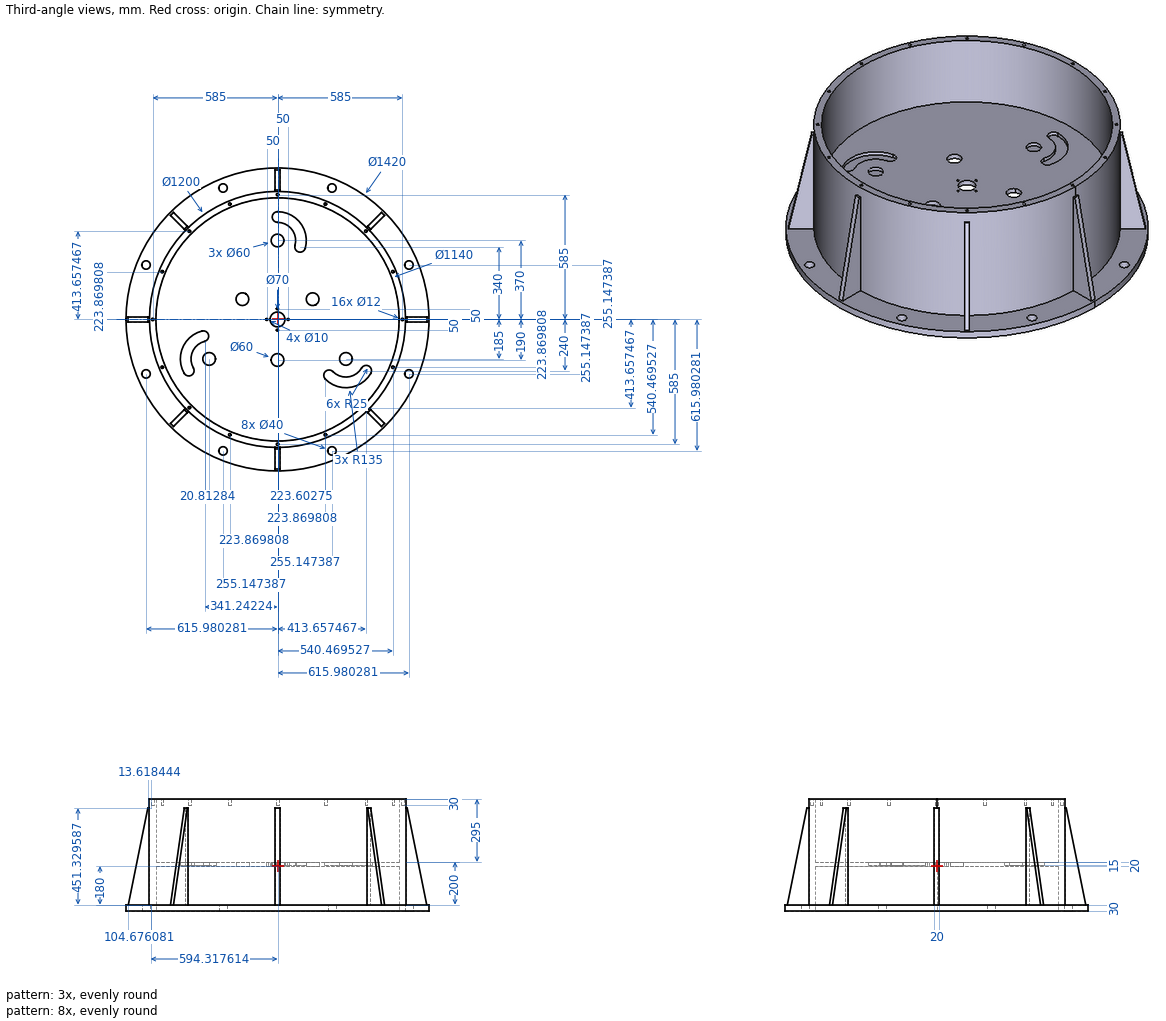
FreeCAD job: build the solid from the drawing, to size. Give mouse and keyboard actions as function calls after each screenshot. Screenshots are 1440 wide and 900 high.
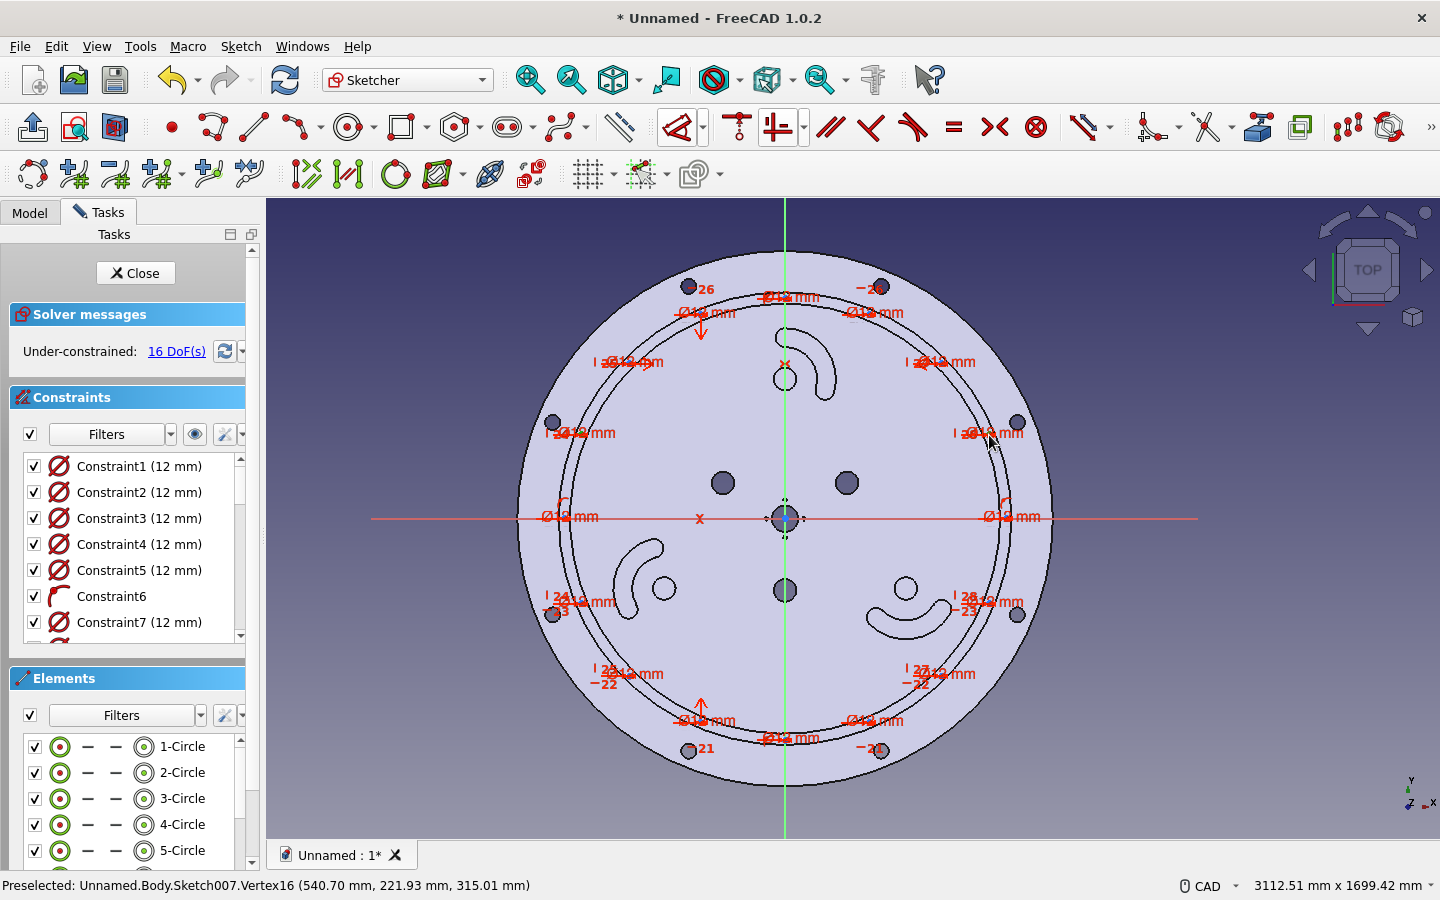
click(785, 686)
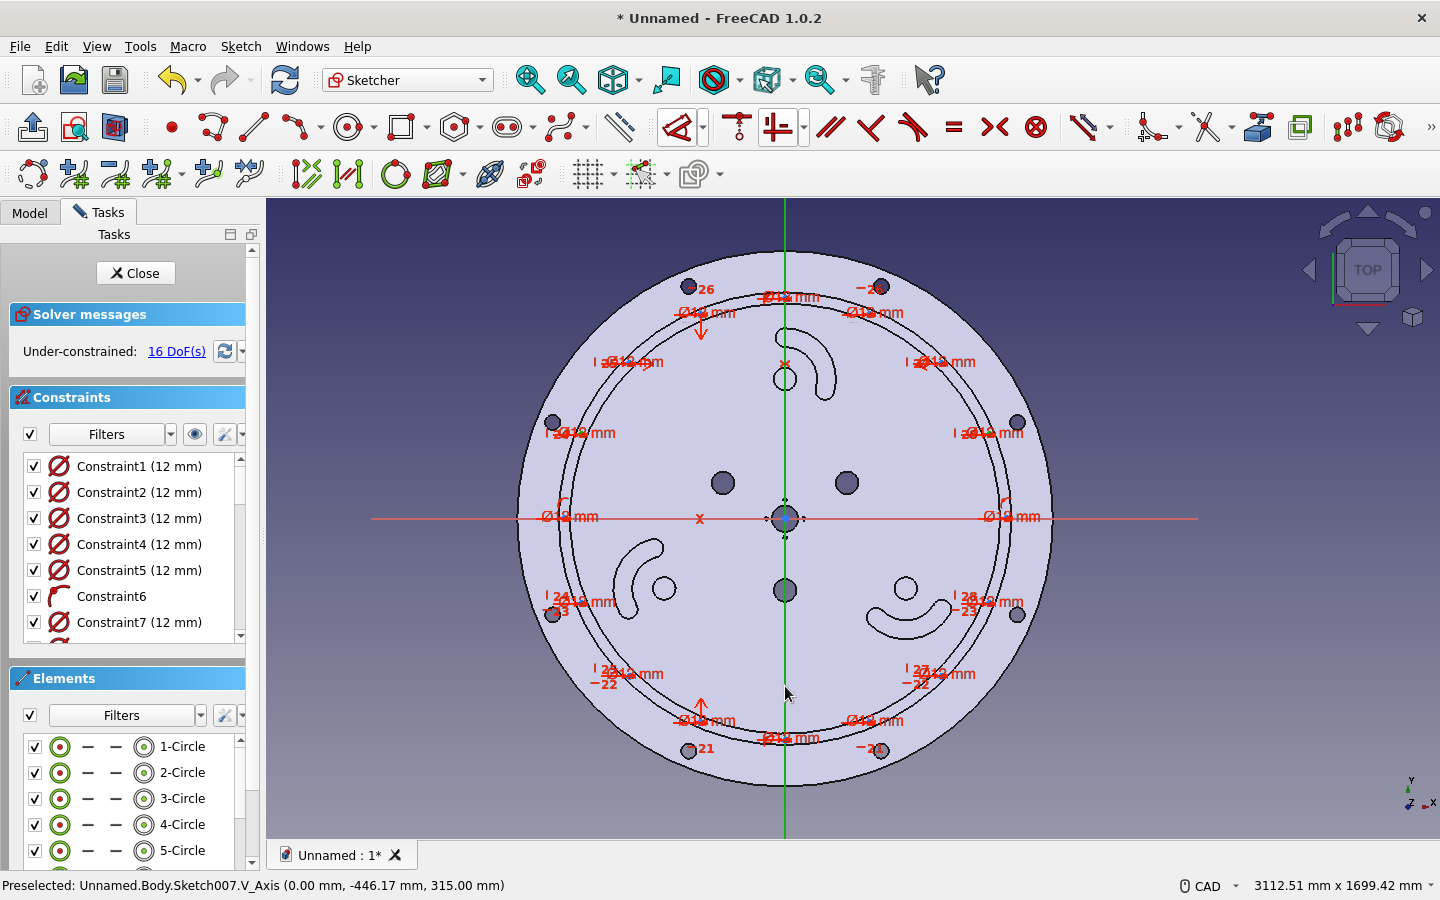
key(s)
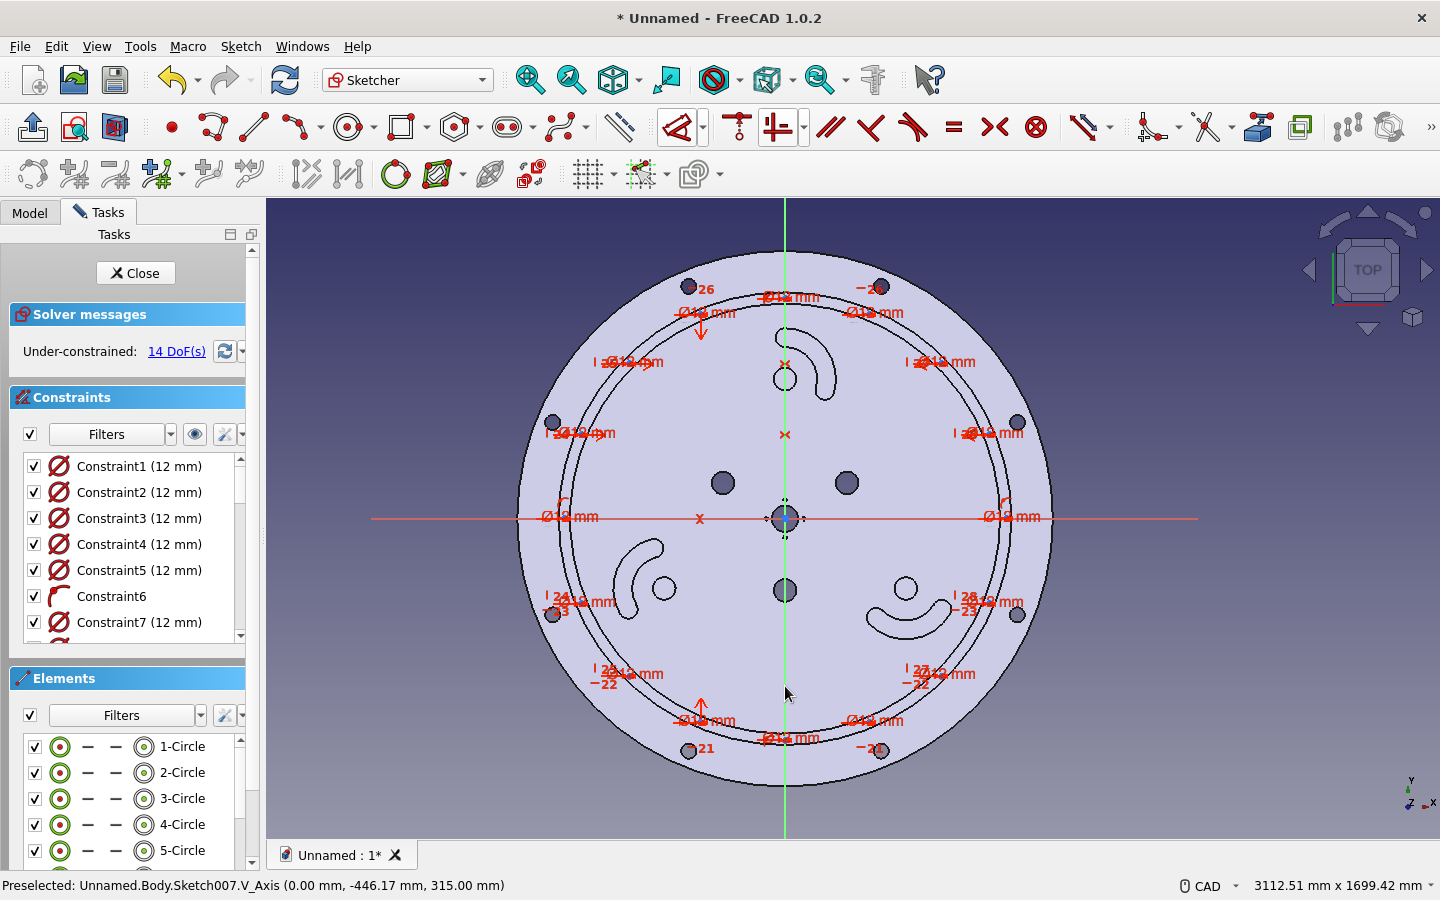
click(1006, 519)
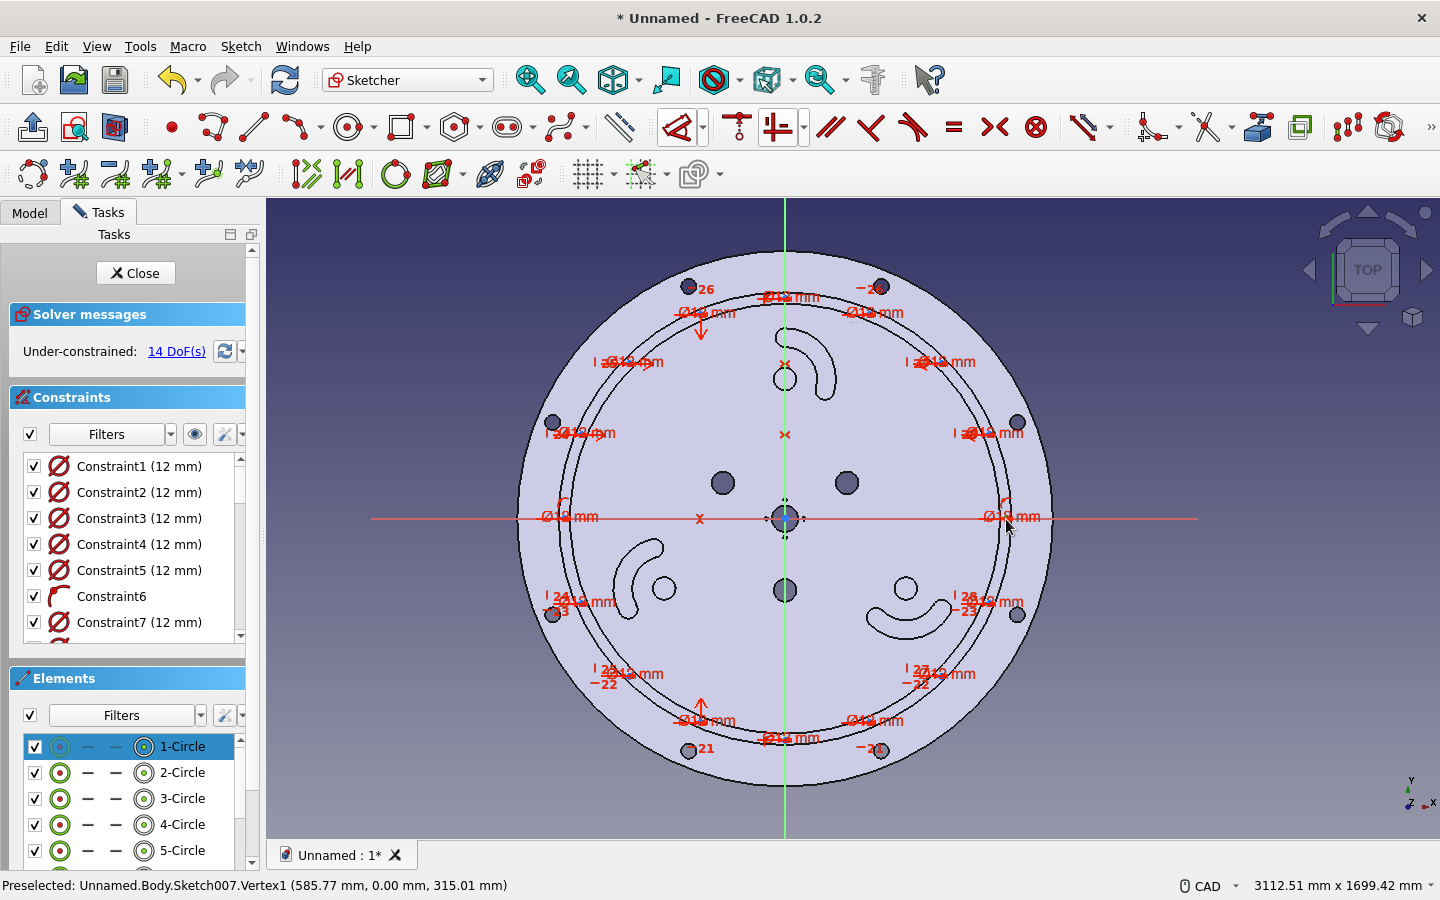
key(l)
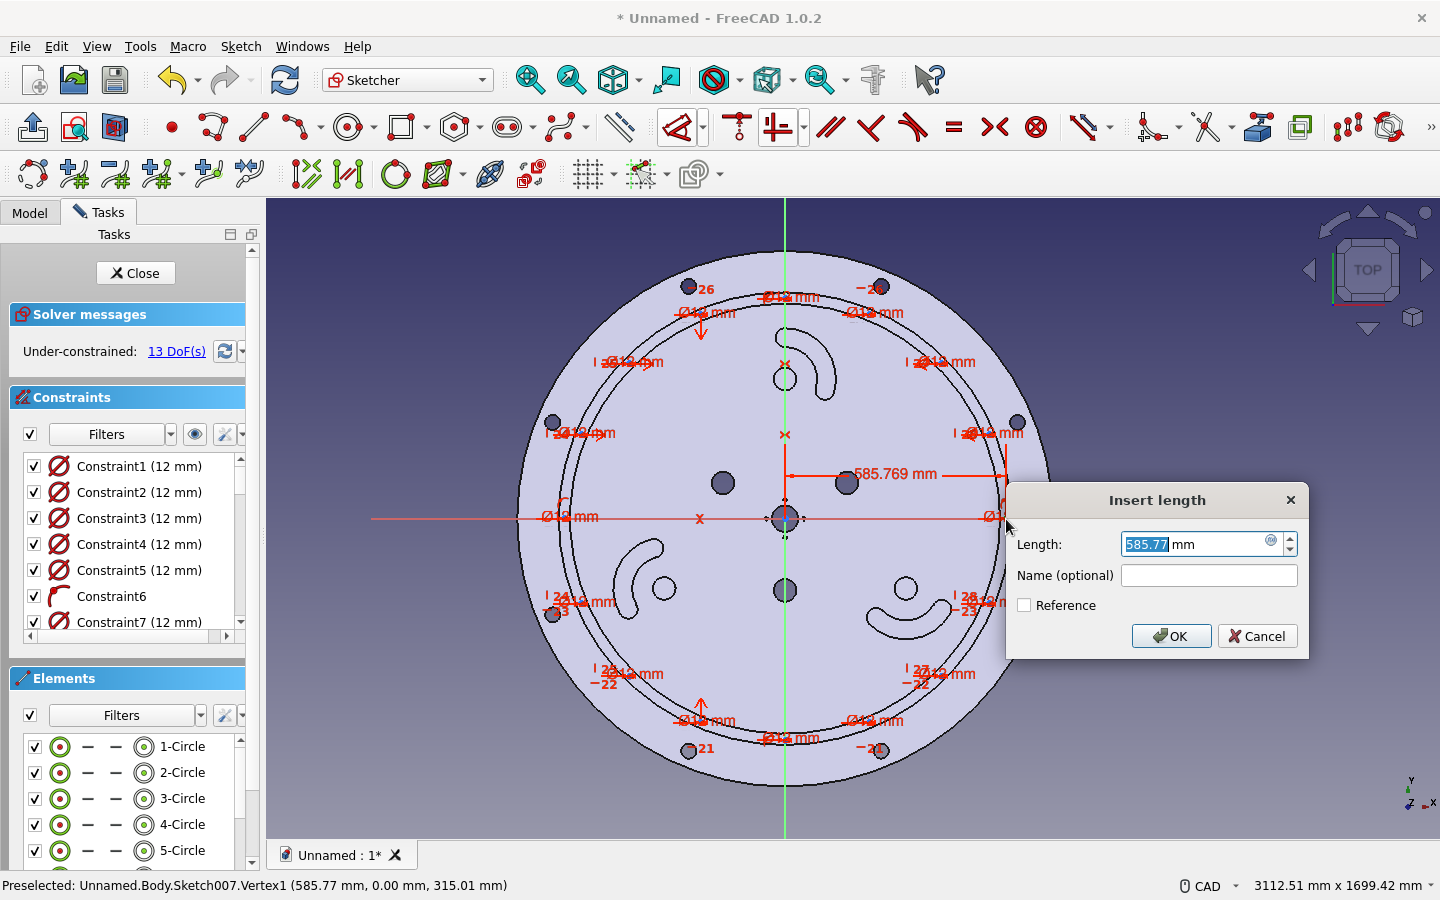
text(585)
key(Return)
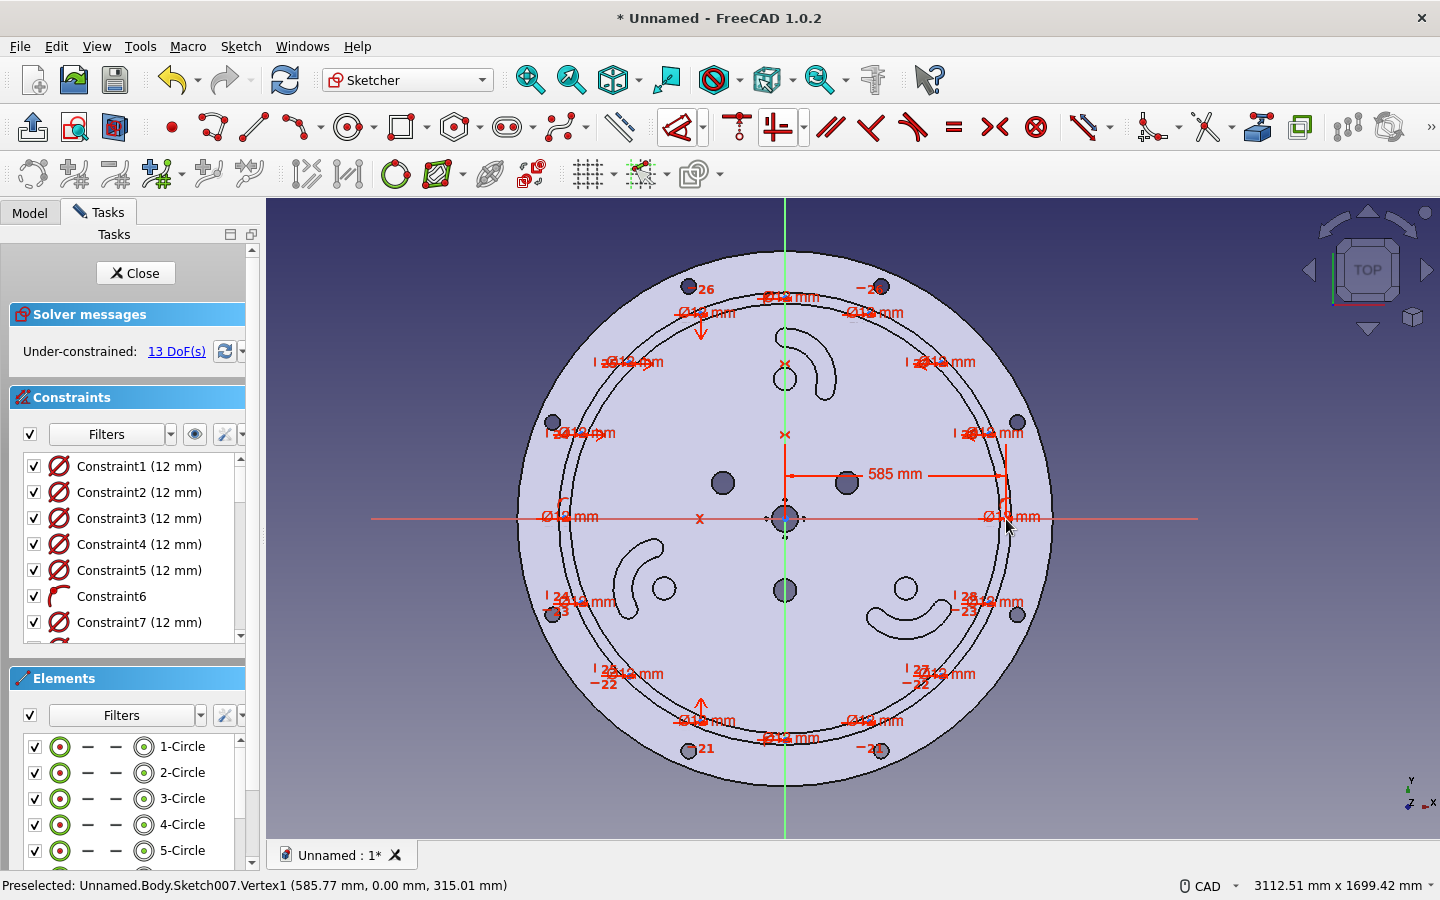
click(785, 740)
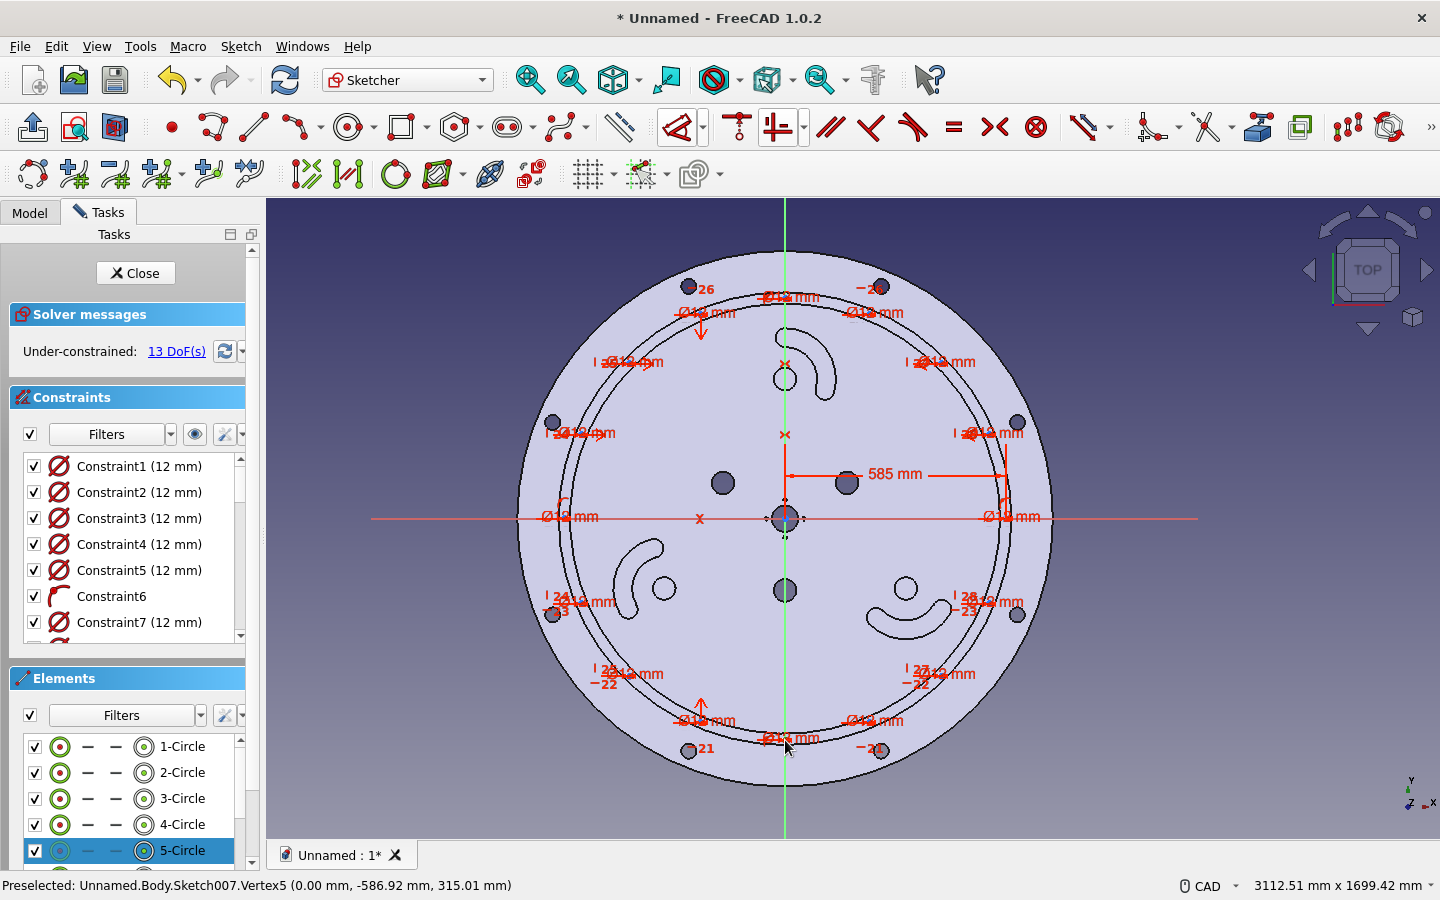
key(i)